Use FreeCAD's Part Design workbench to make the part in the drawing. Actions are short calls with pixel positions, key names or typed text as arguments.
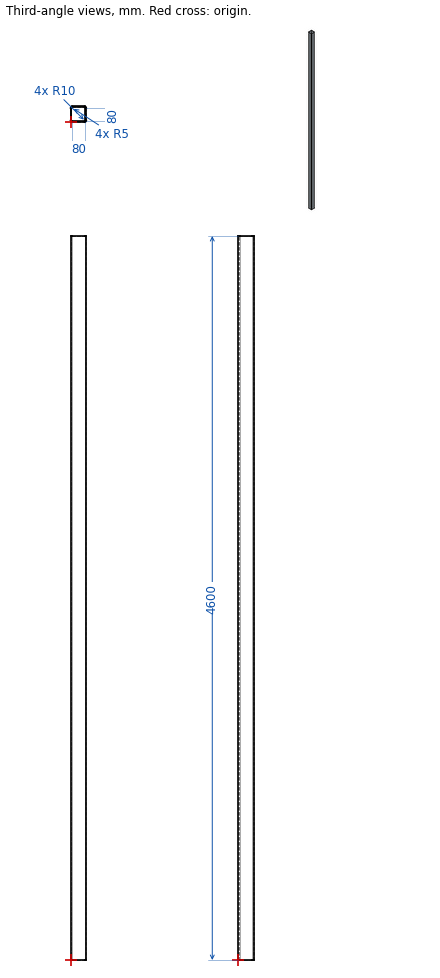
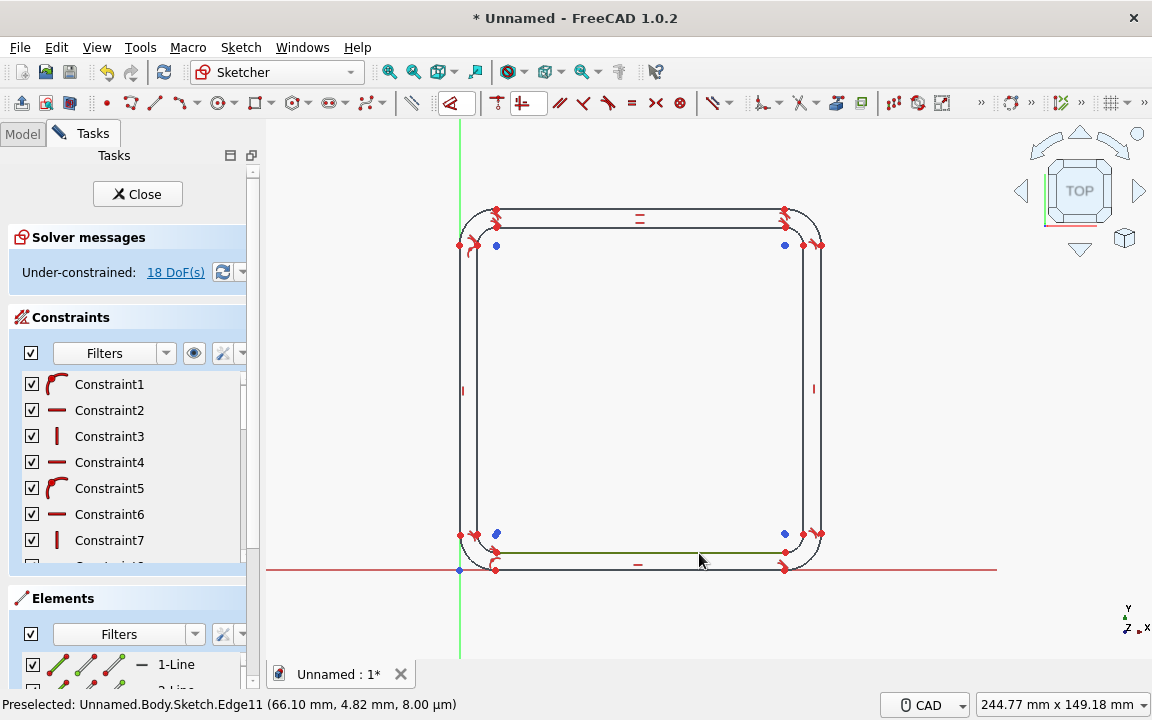
click(483, 547)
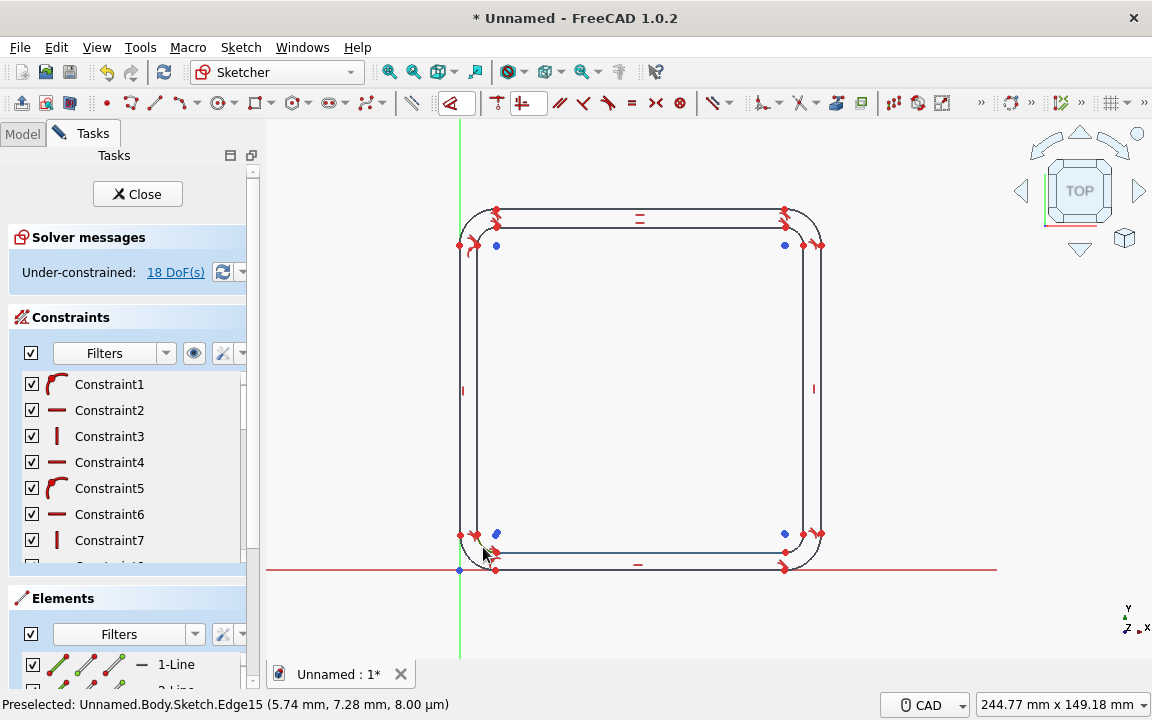
click(608, 104)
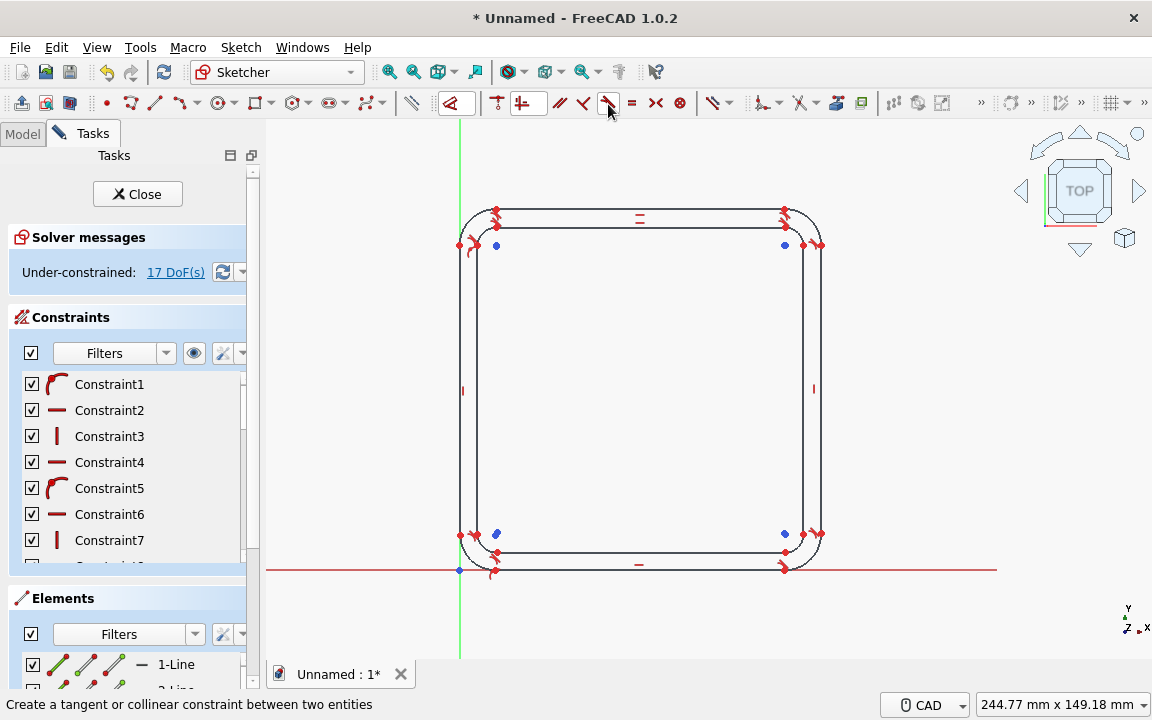
click(477, 448)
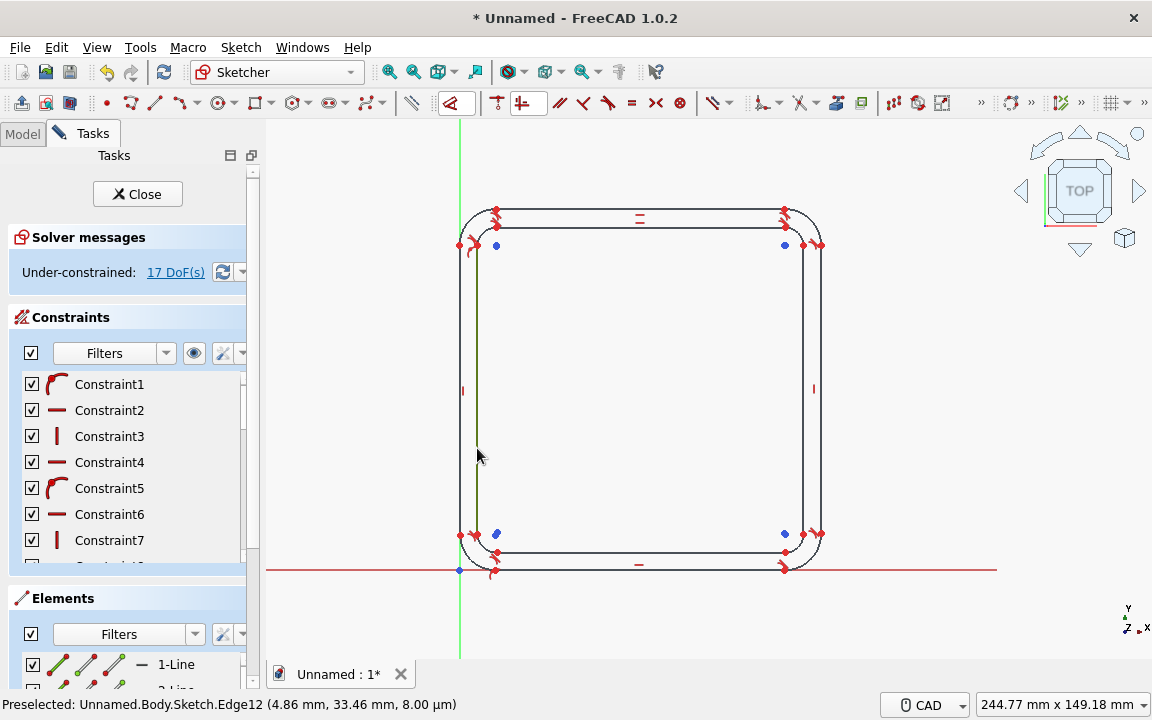
click(484, 547)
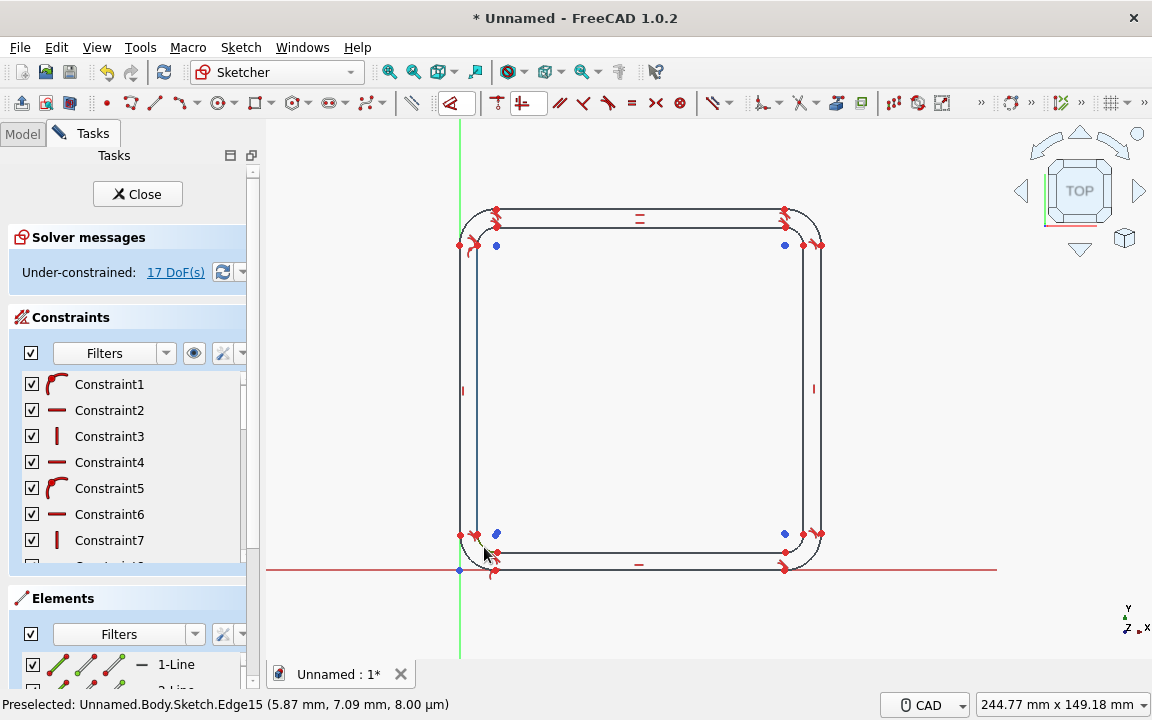
click(608, 104)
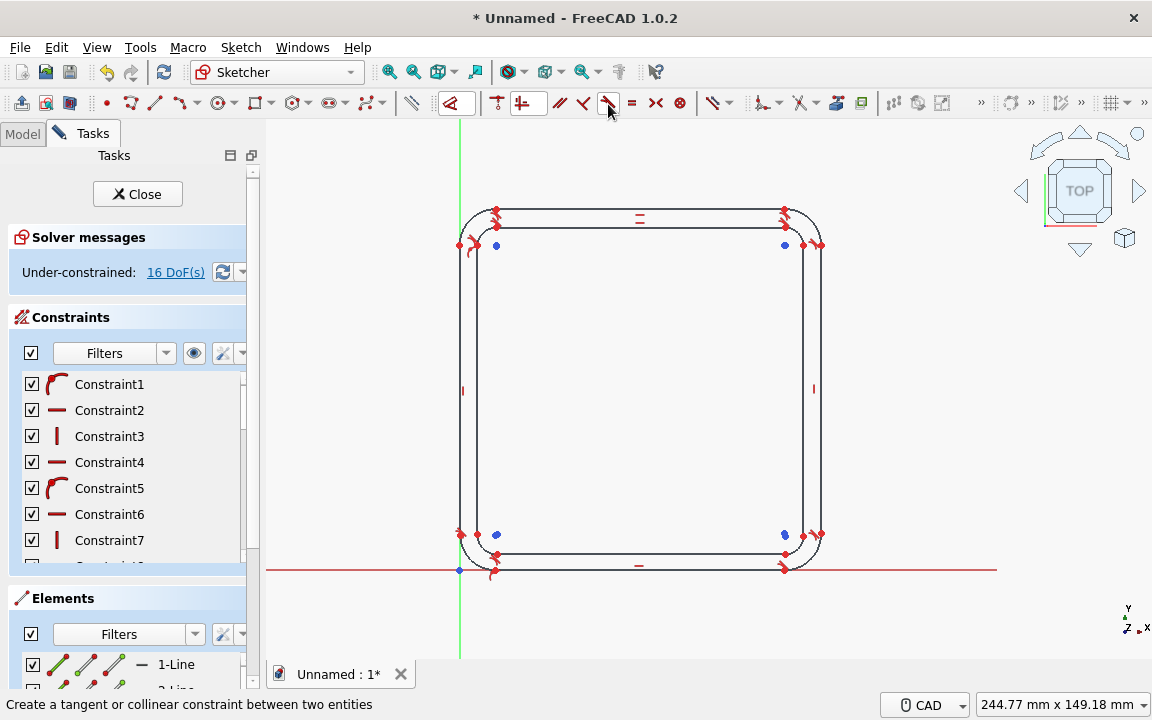
click(477, 448)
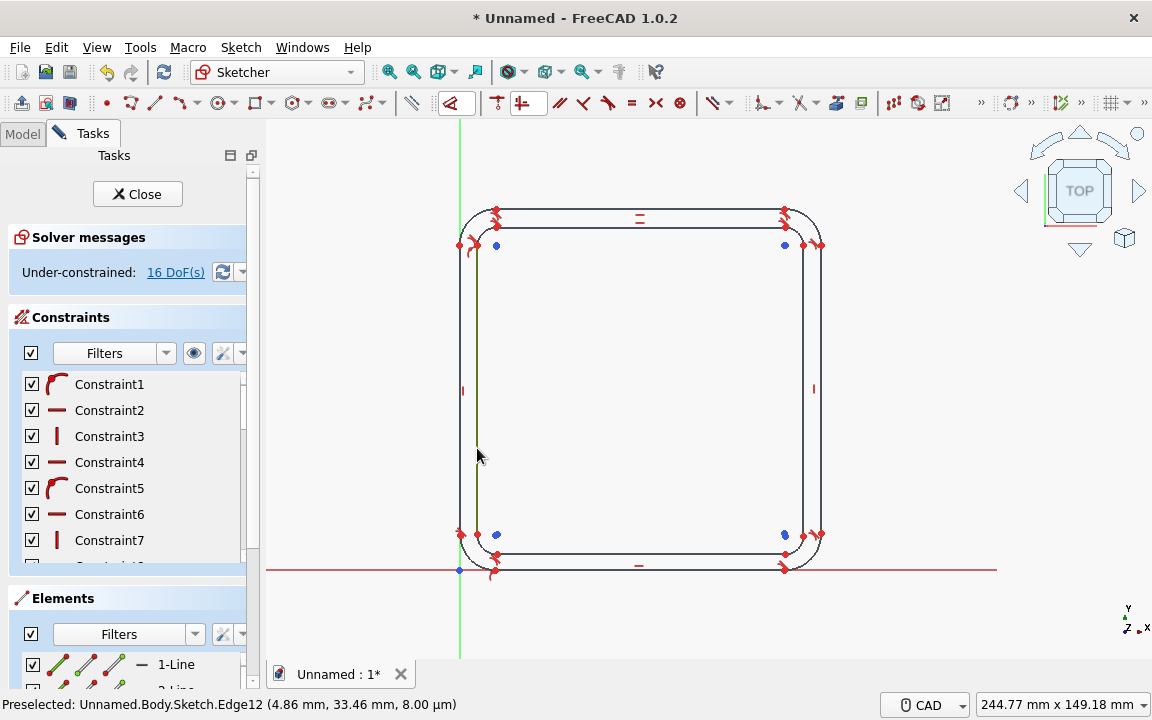
click(483, 233)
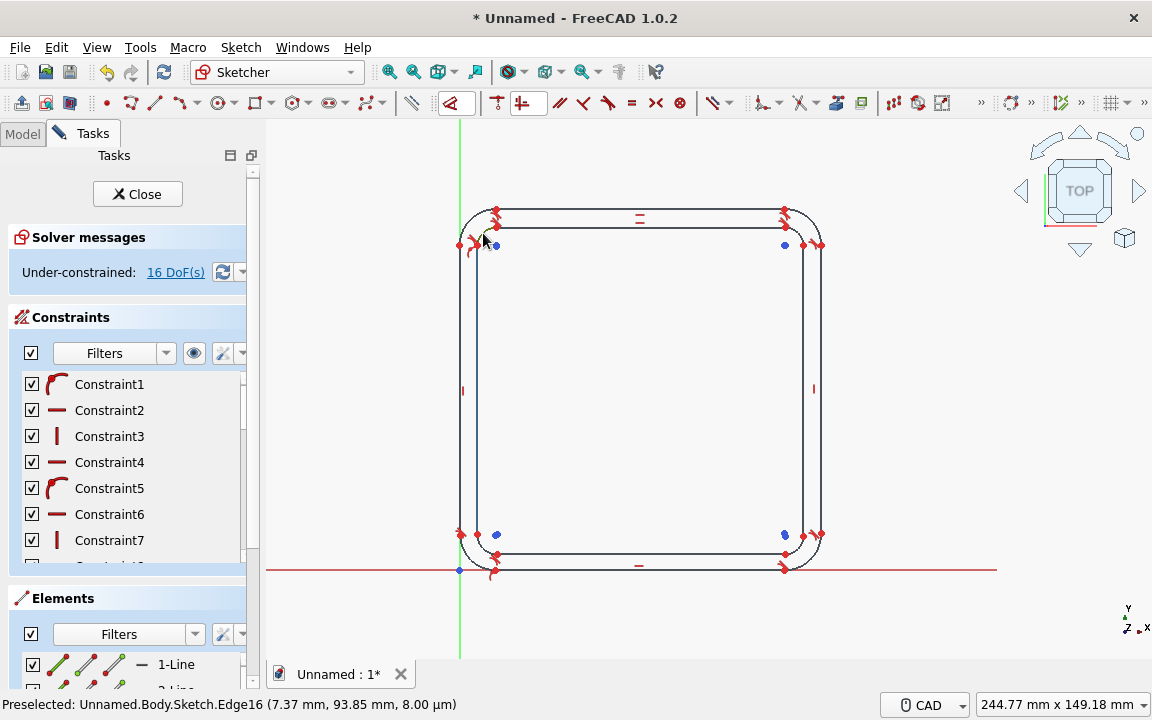
key(t)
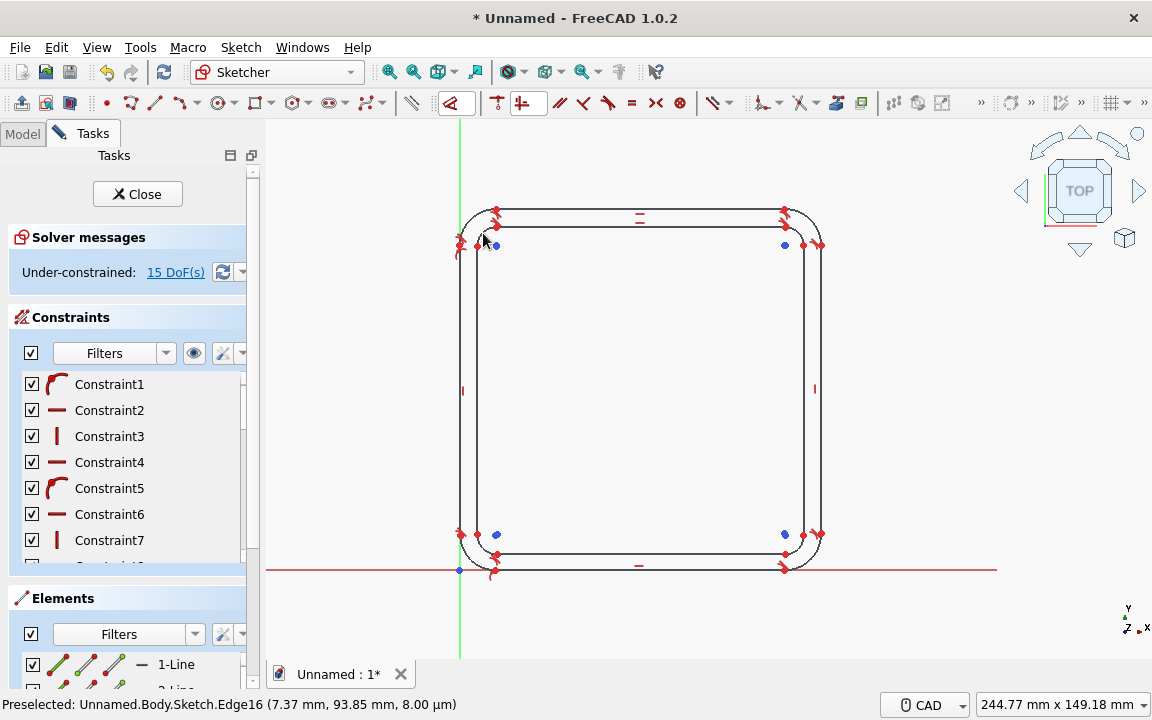
click(460, 333)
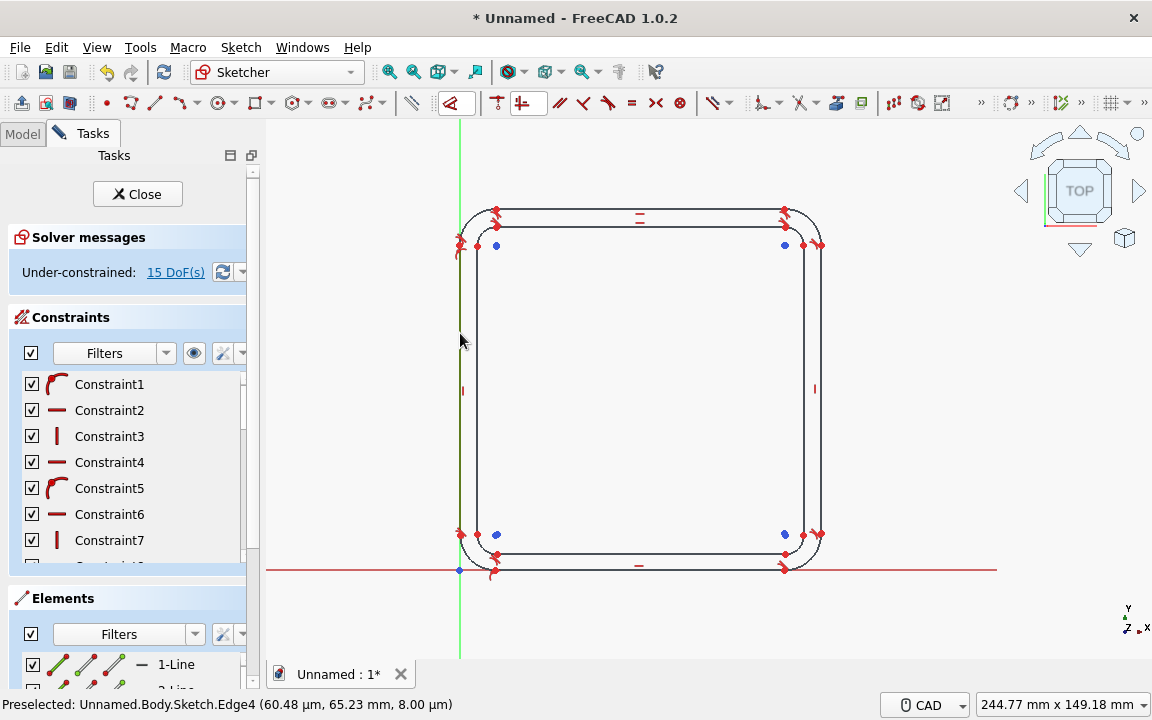
key(v)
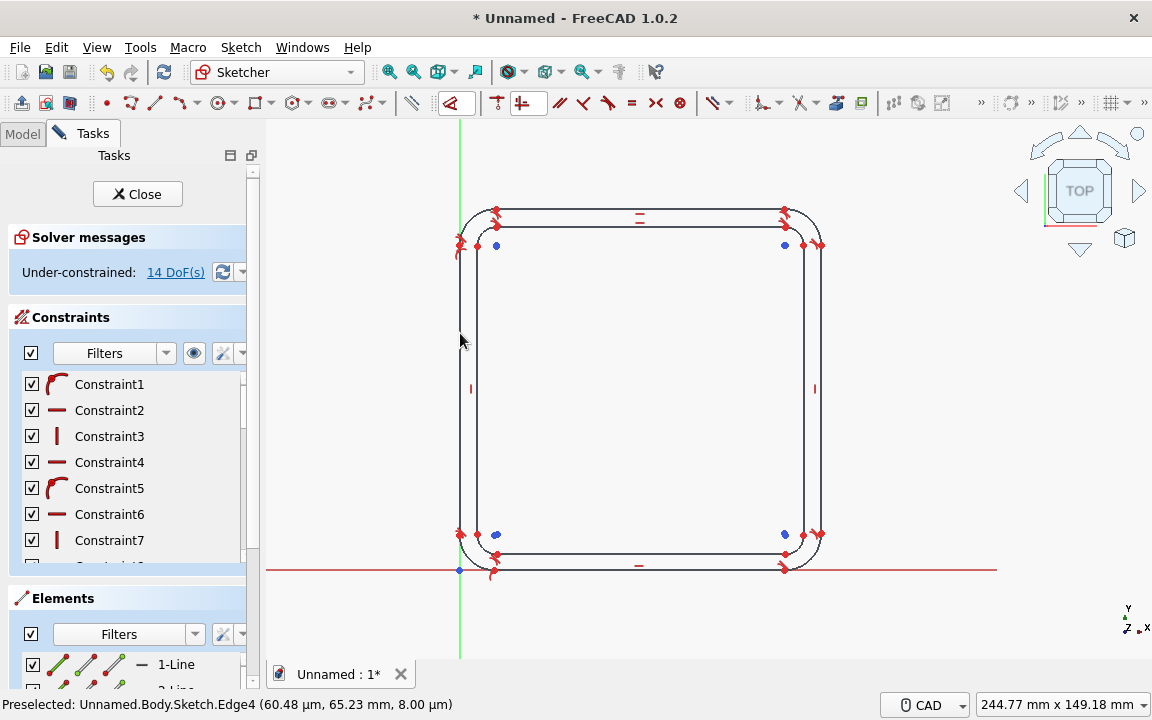
click(817, 229)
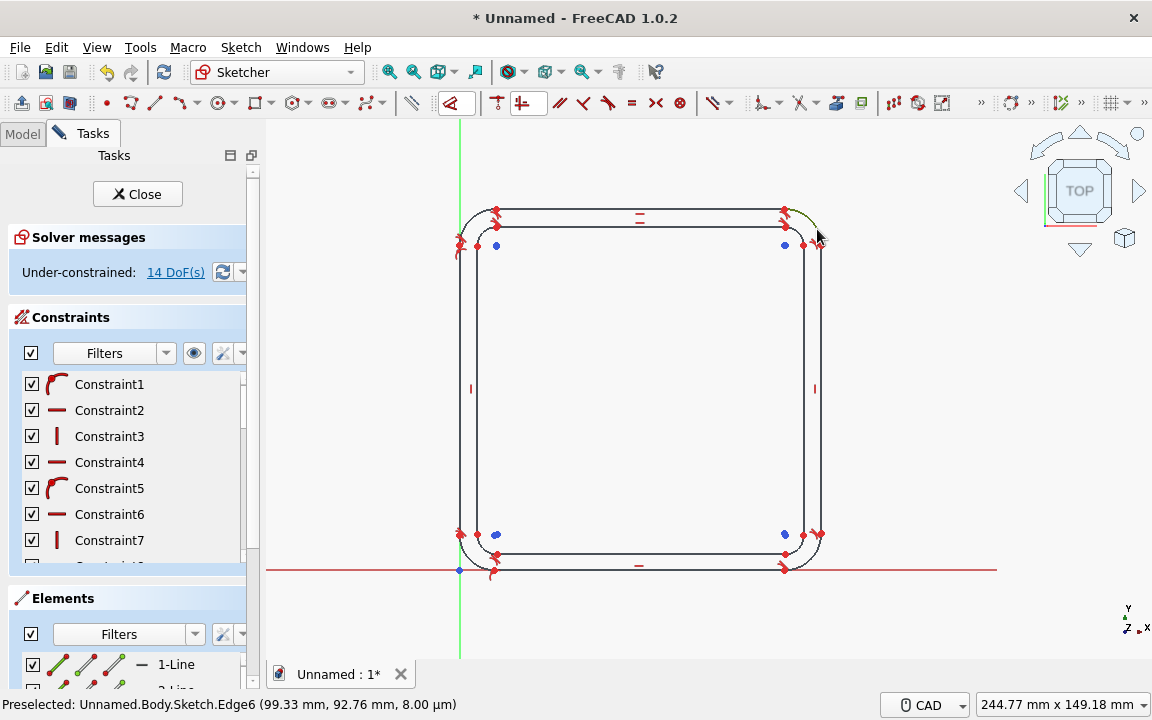
click(798, 233)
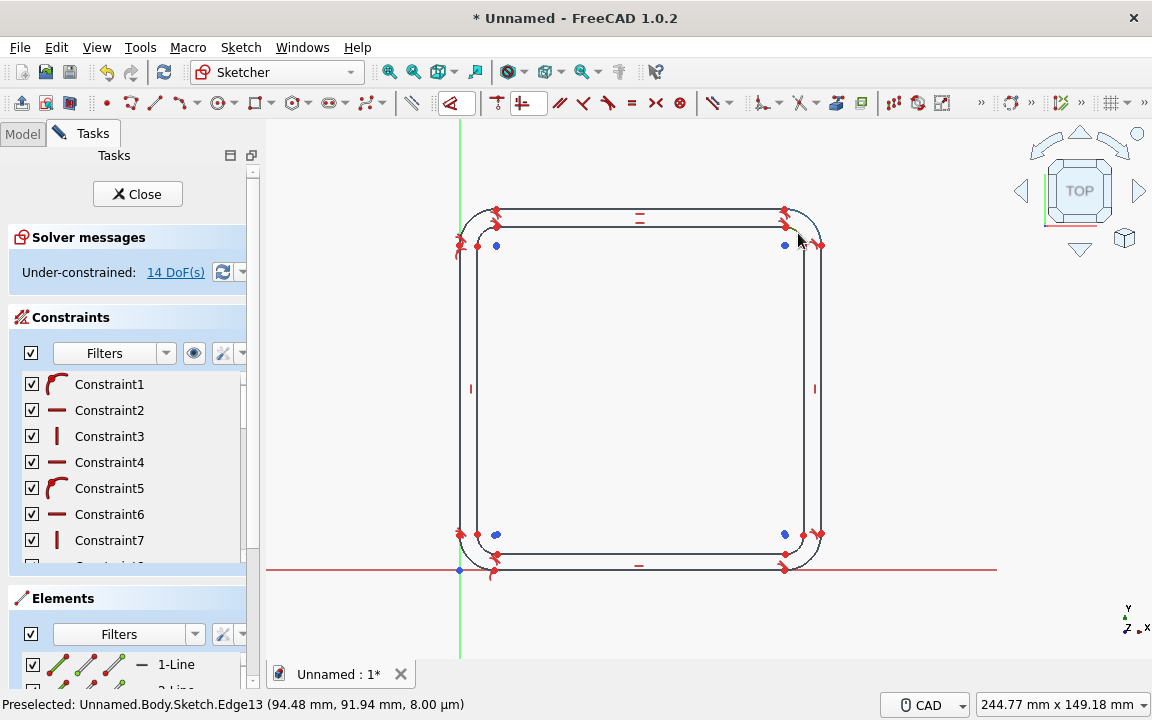
click(498, 104)